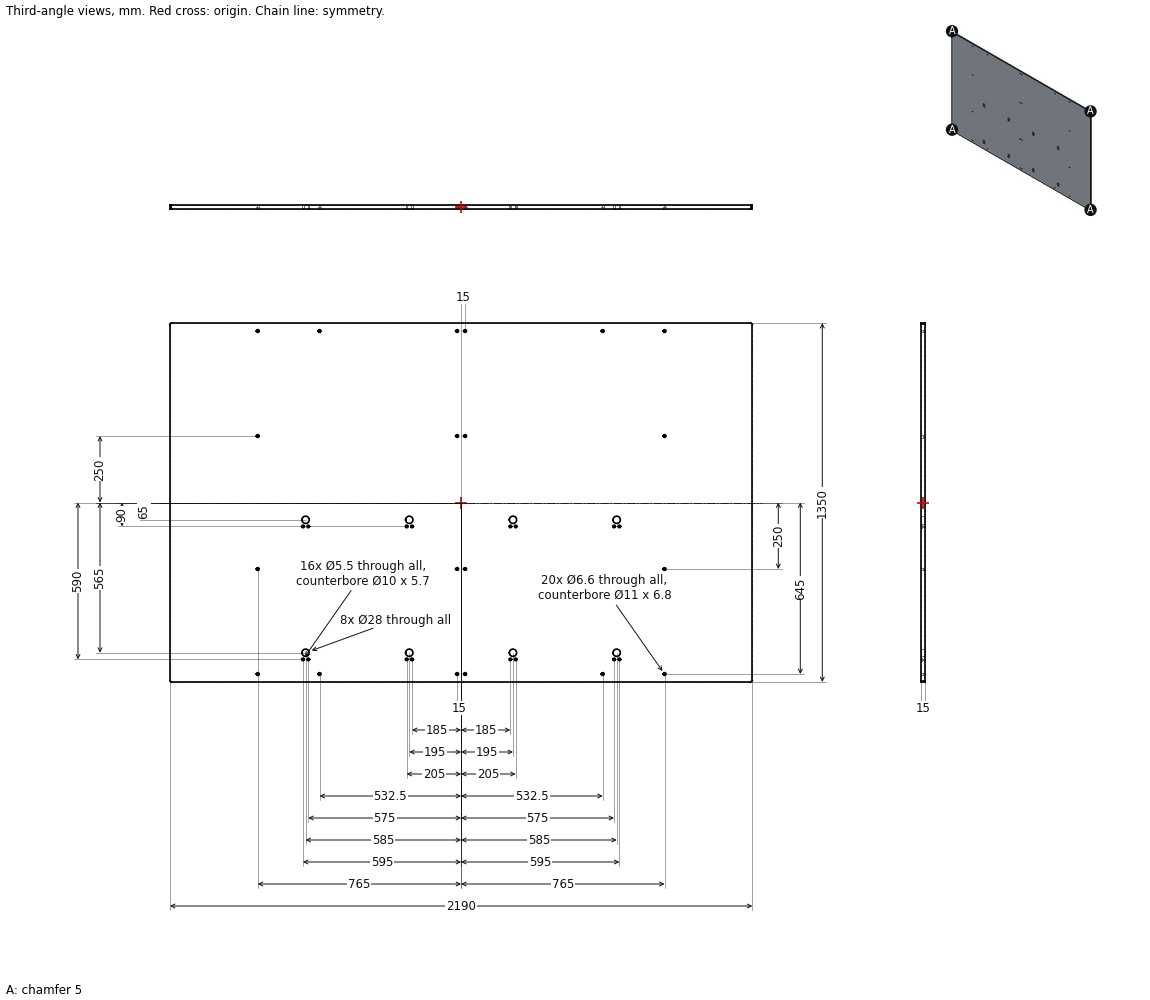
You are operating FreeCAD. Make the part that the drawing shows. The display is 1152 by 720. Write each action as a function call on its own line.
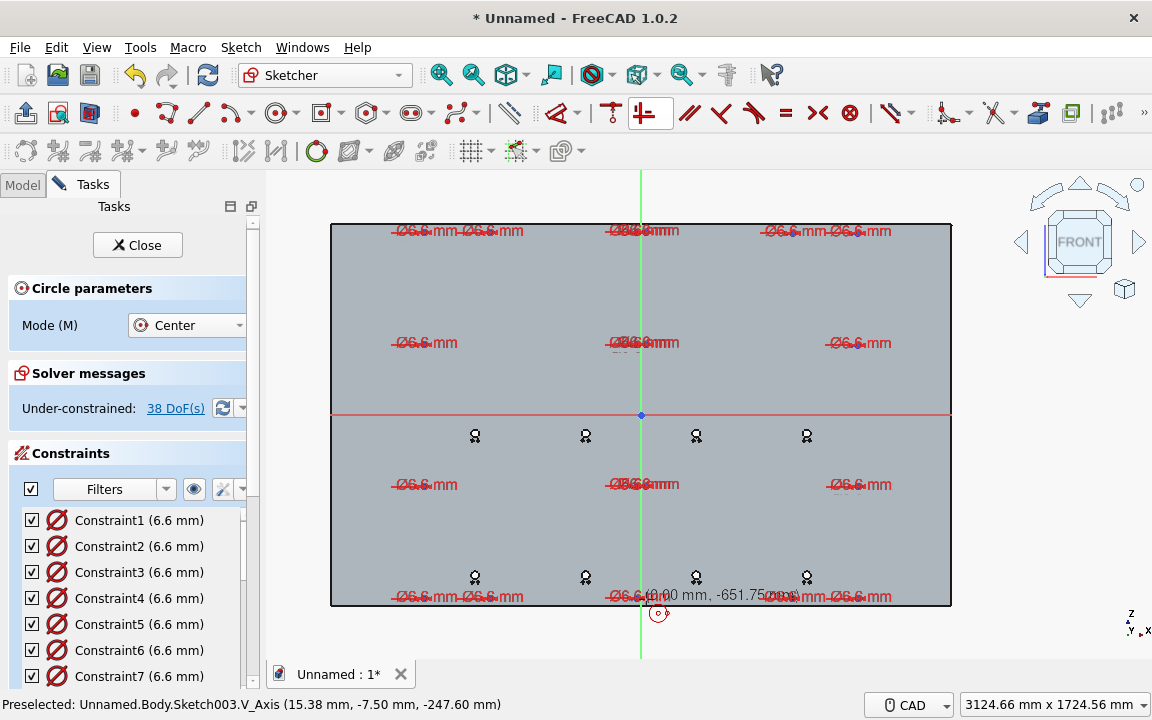
scroll(645, 598, up, 7)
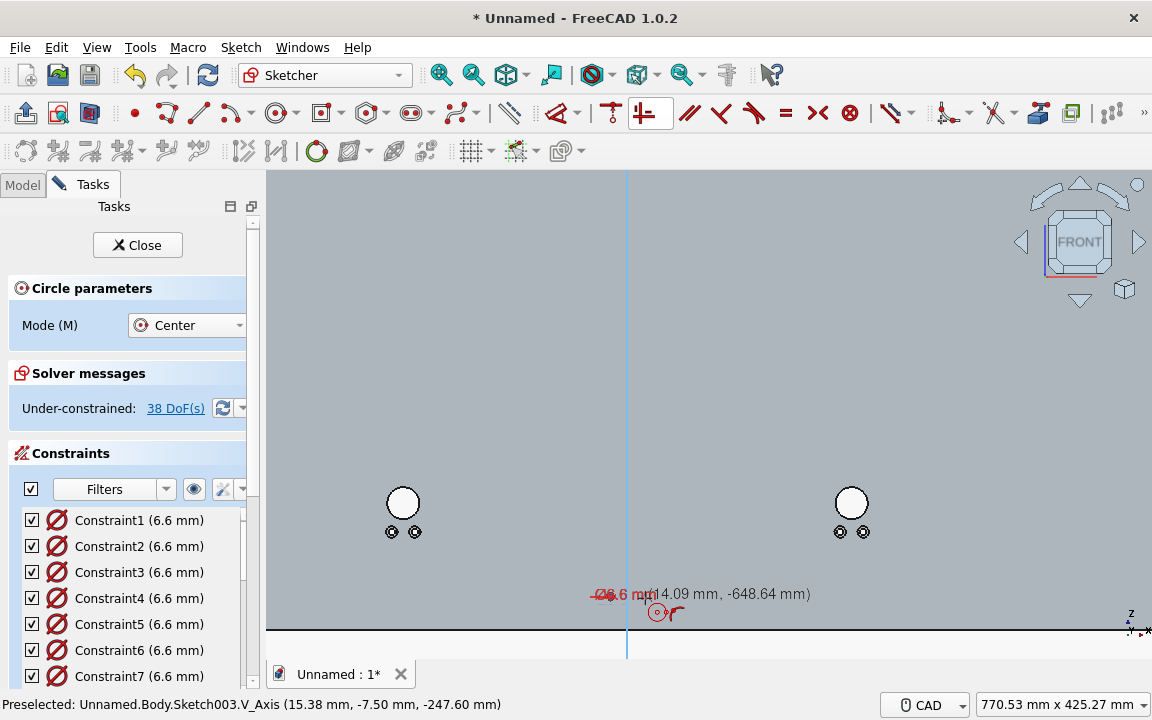
click(645, 595)
move(647, 593)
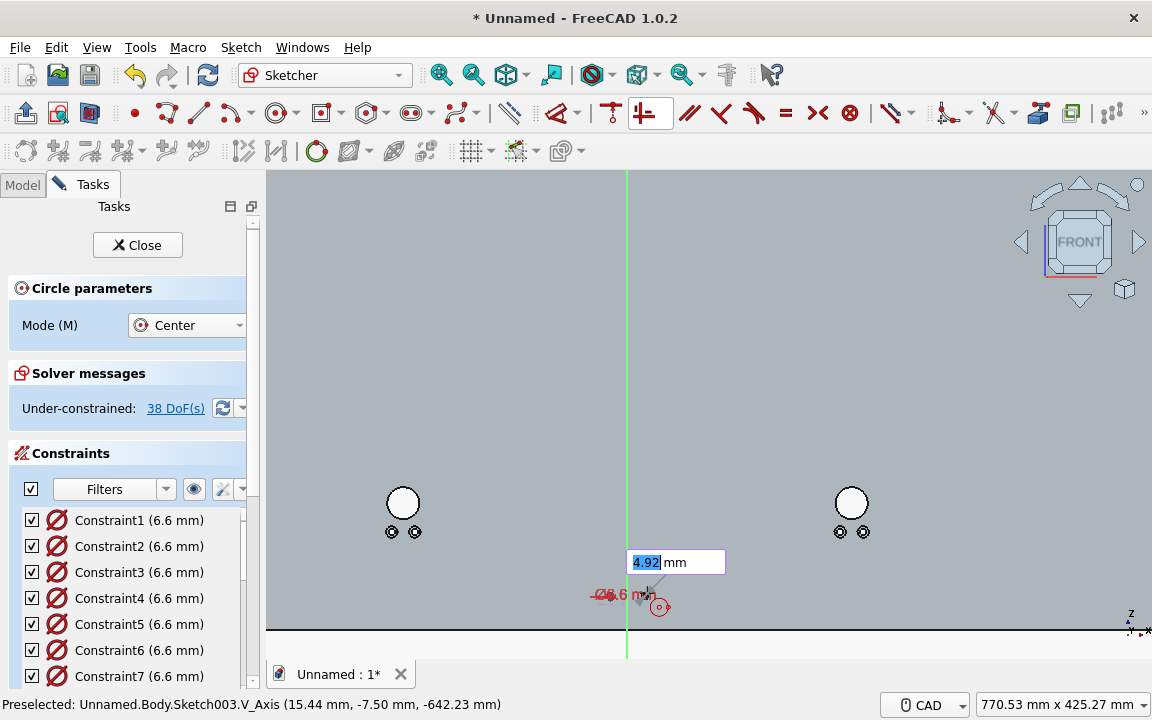
text(6.6)
key(Return)
key(Escape)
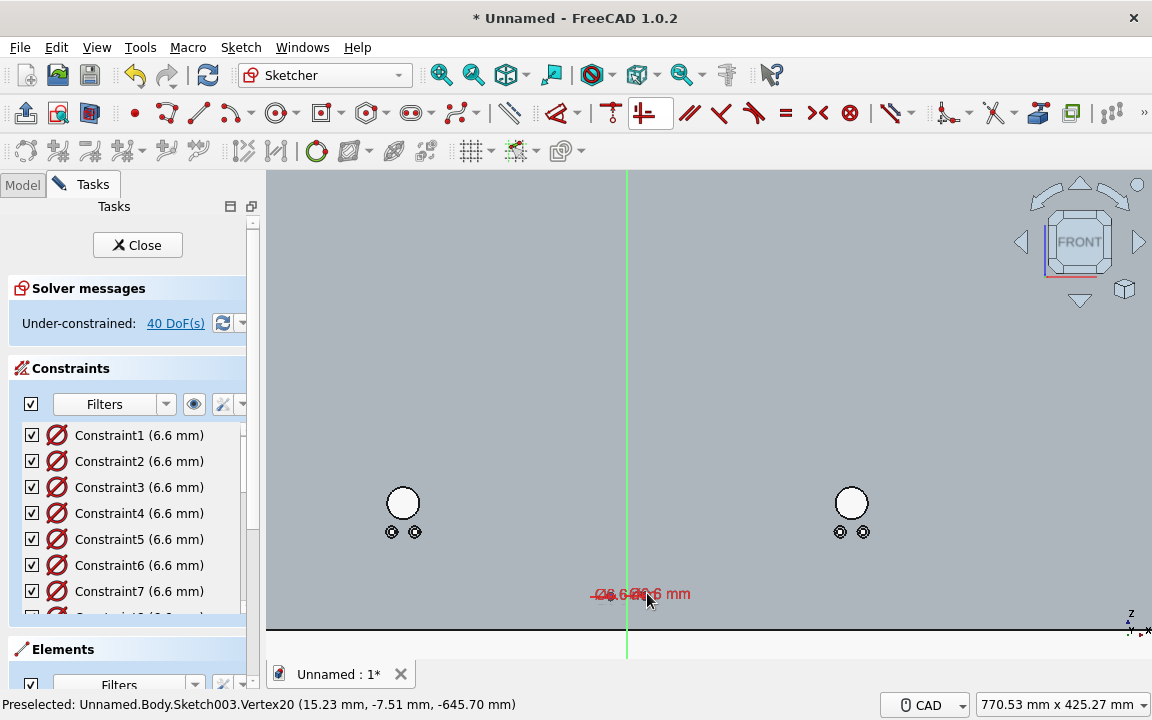
scroll(644, 556, down, 8)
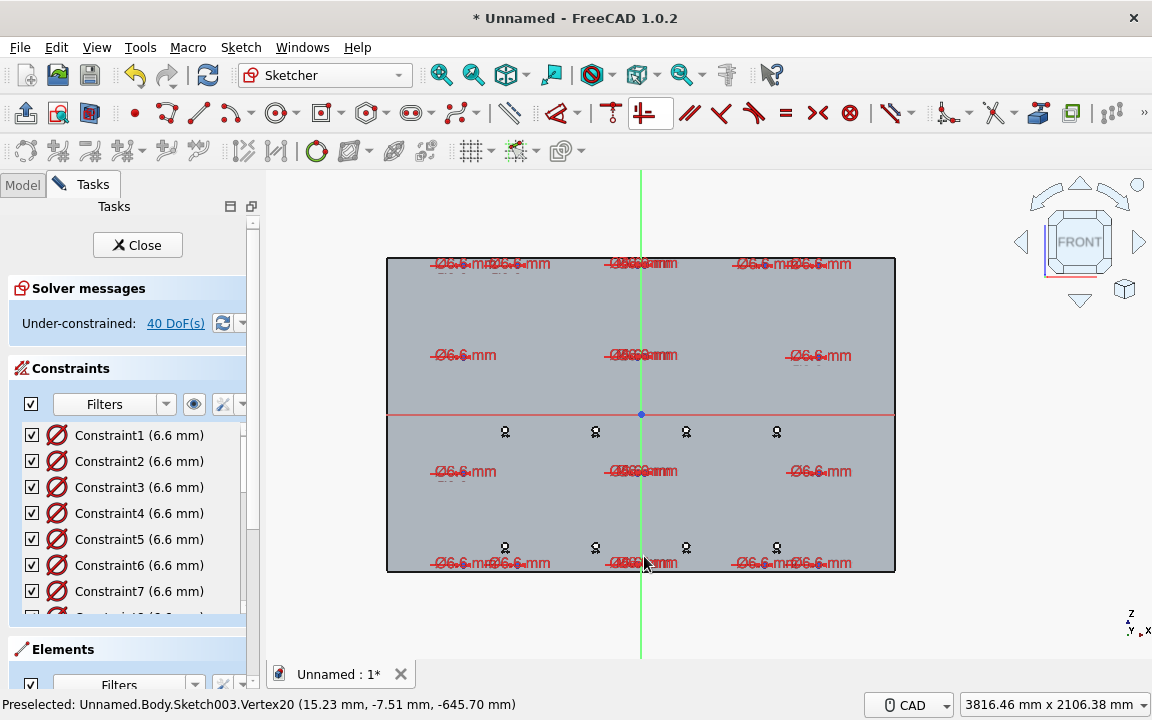
click(819, 565)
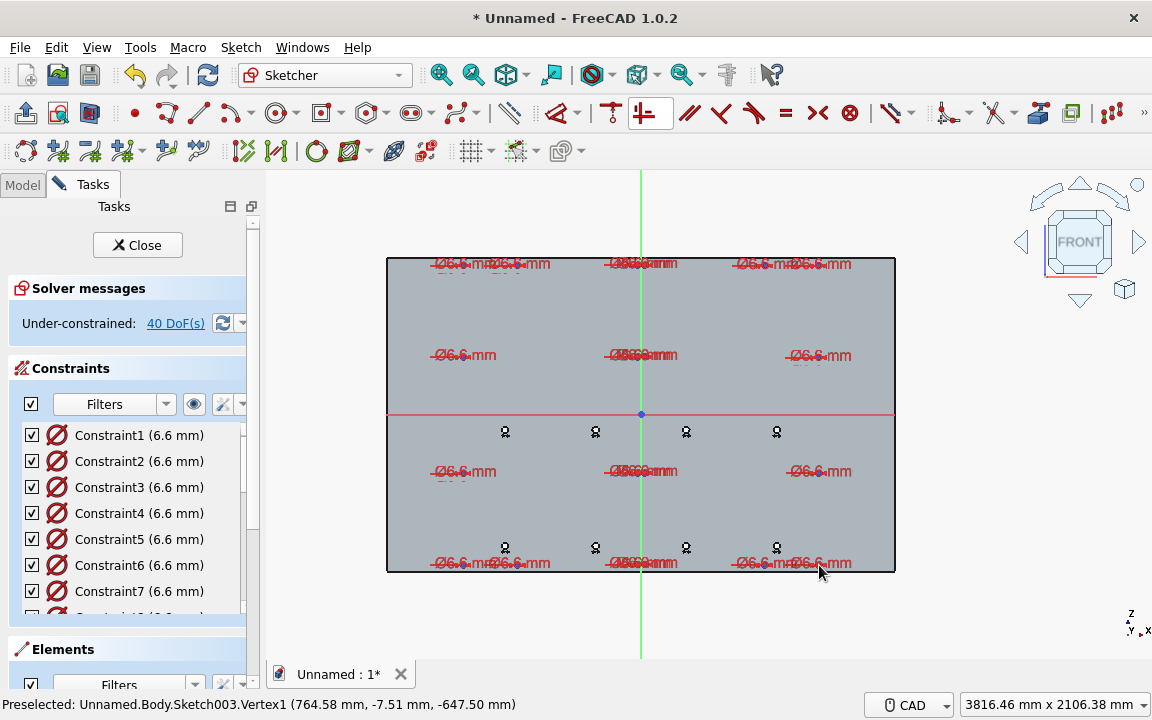
click(764, 565)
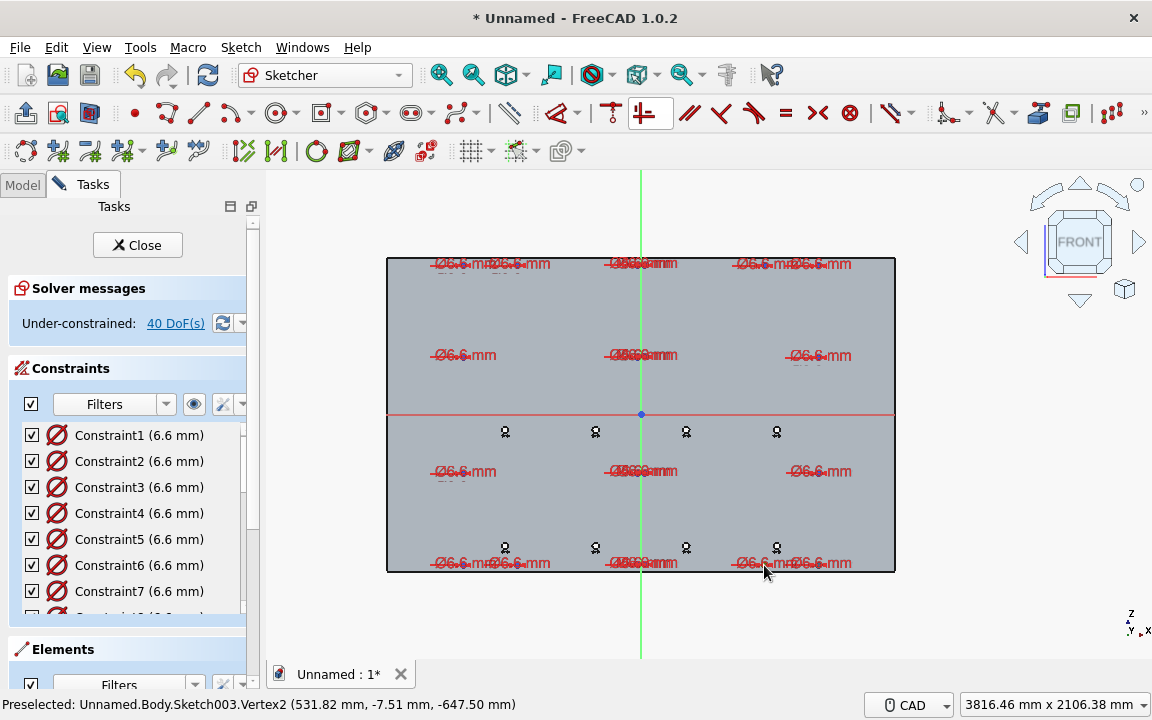
key(h)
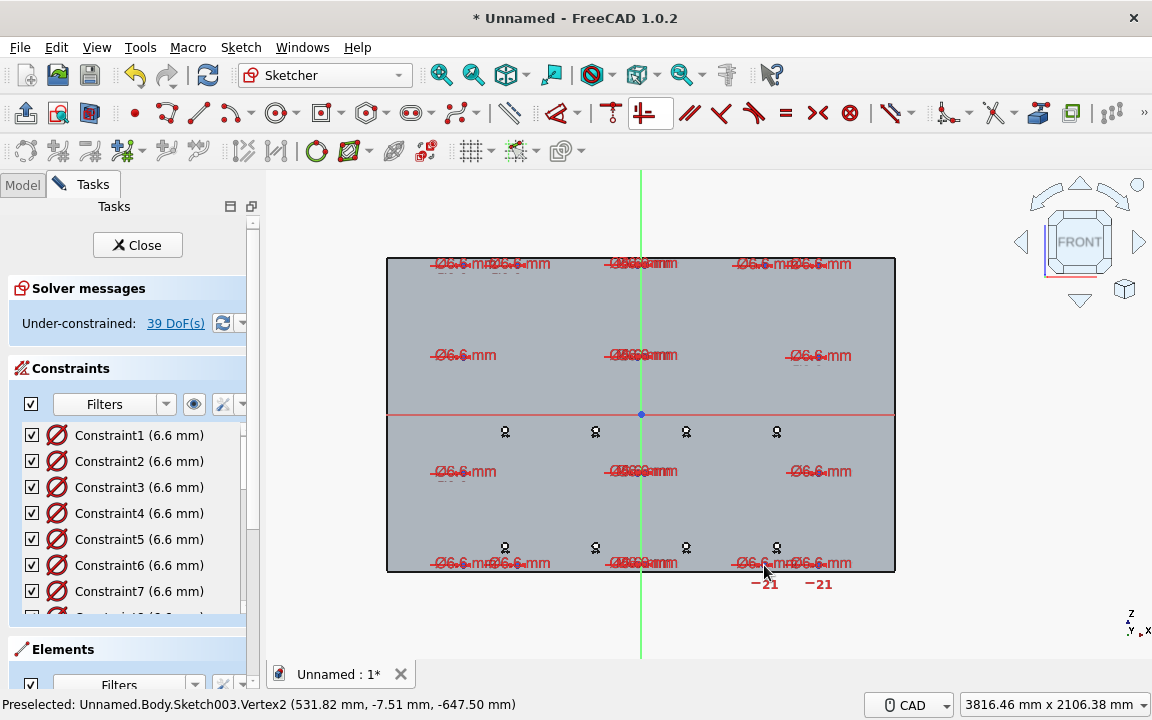
click(819, 565)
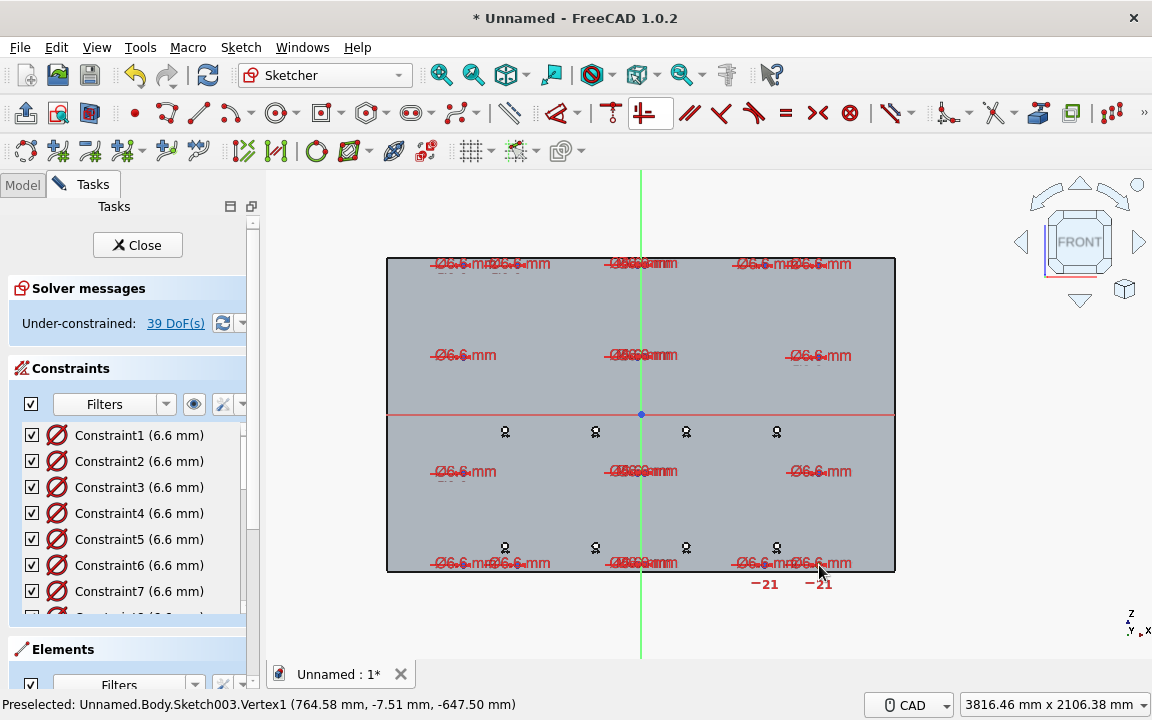
click(819, 473)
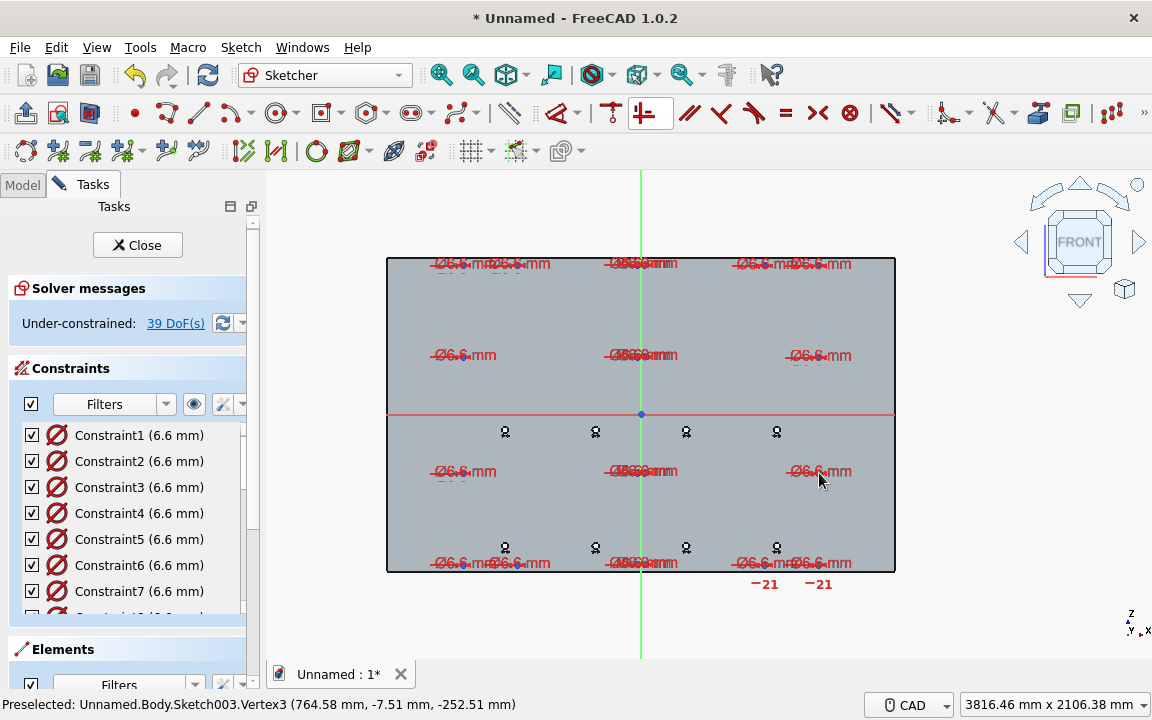
key(v)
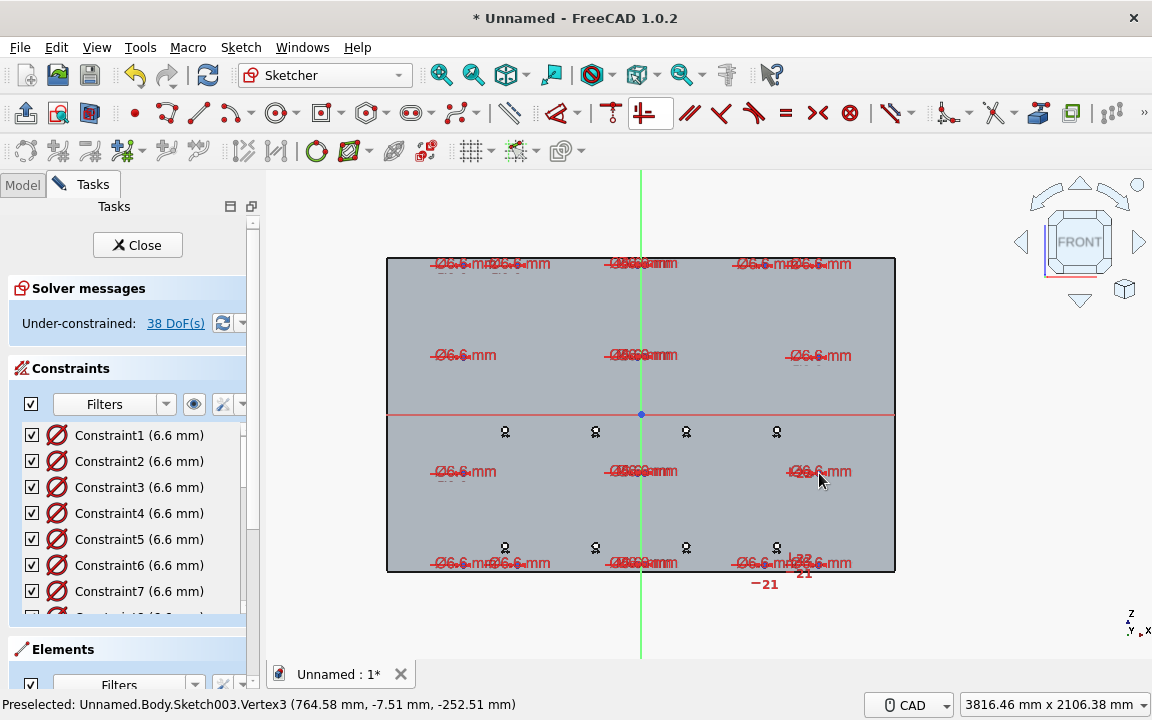
click(764, 565)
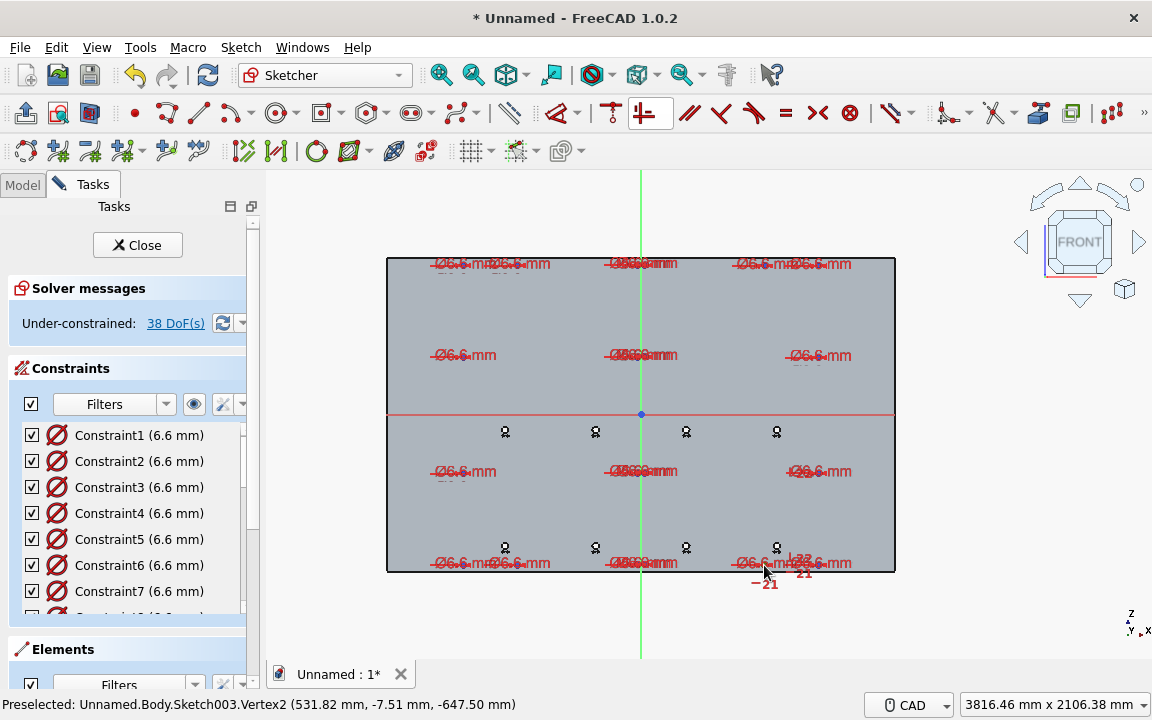
scroll(638, 565, up, 3)